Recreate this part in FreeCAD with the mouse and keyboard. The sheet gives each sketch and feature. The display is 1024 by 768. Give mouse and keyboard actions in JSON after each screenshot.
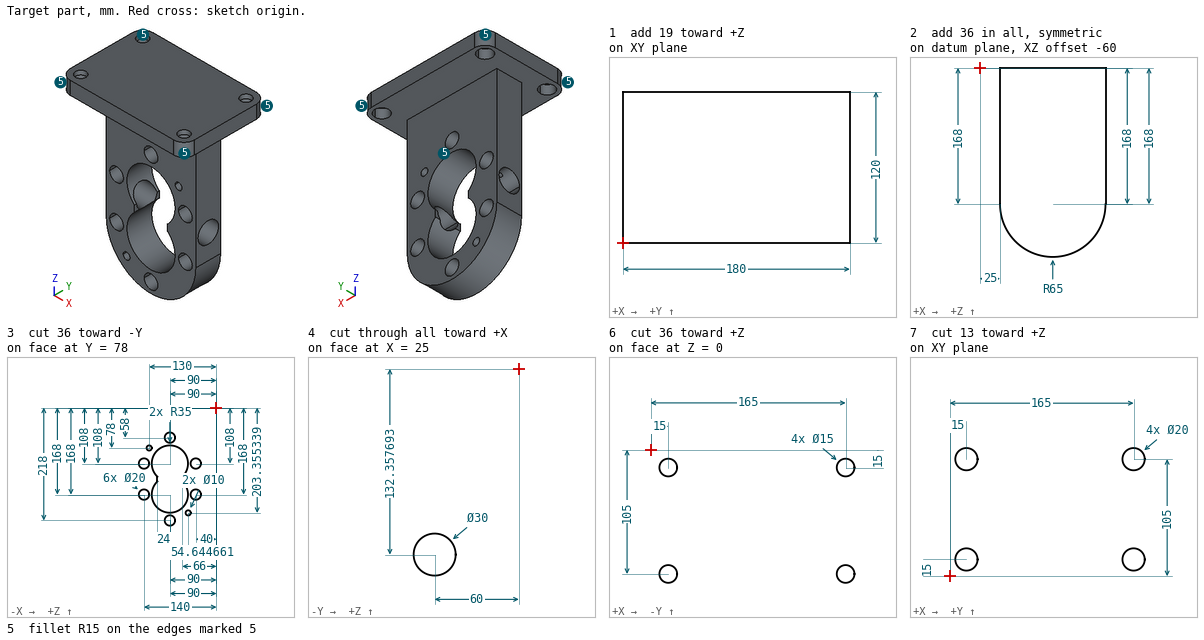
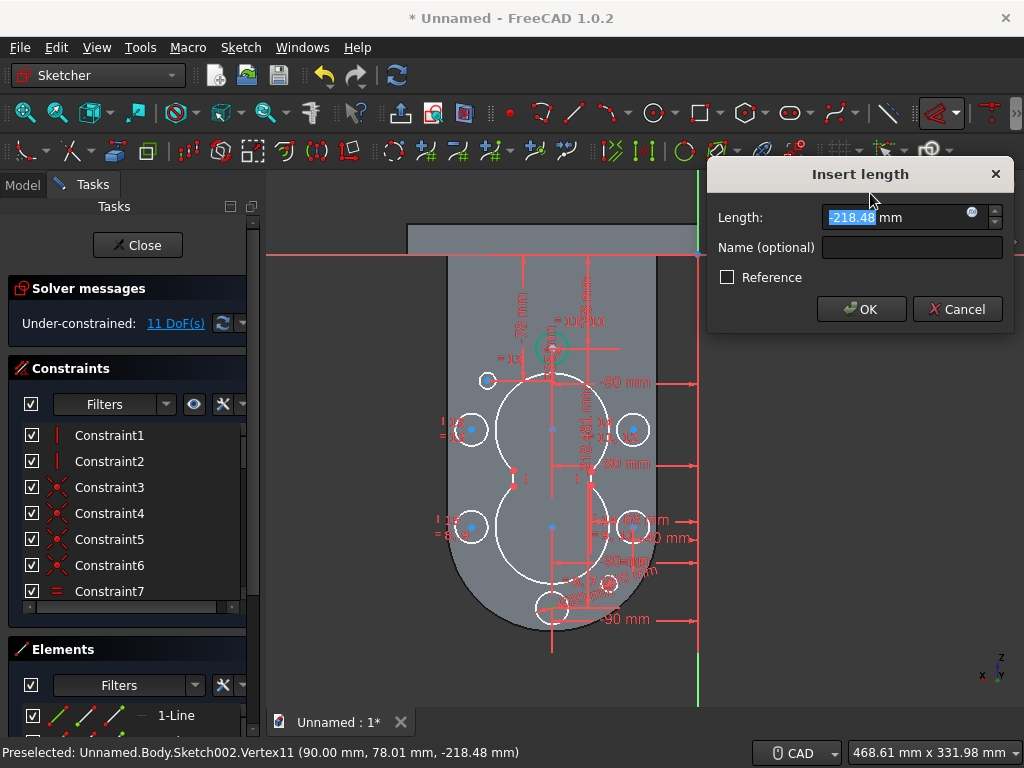
{"action": "type", "text": "-218"}
{"action": "key", "text": "Return"}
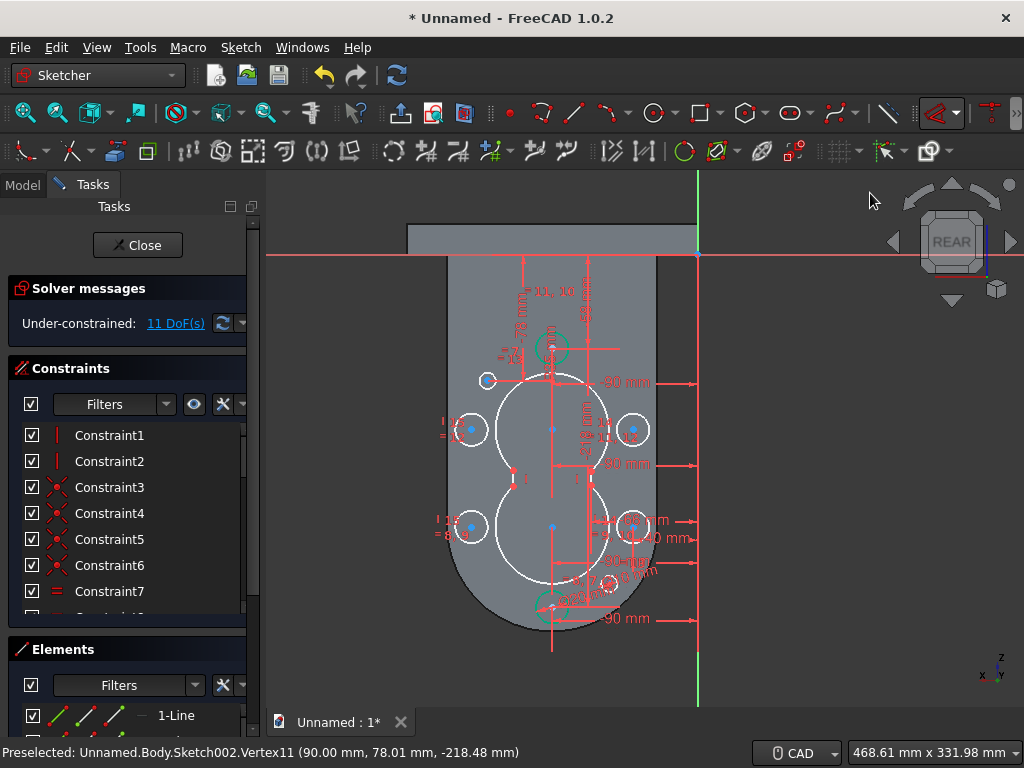
{"action": "left_click", "coordinate": [472, 527]}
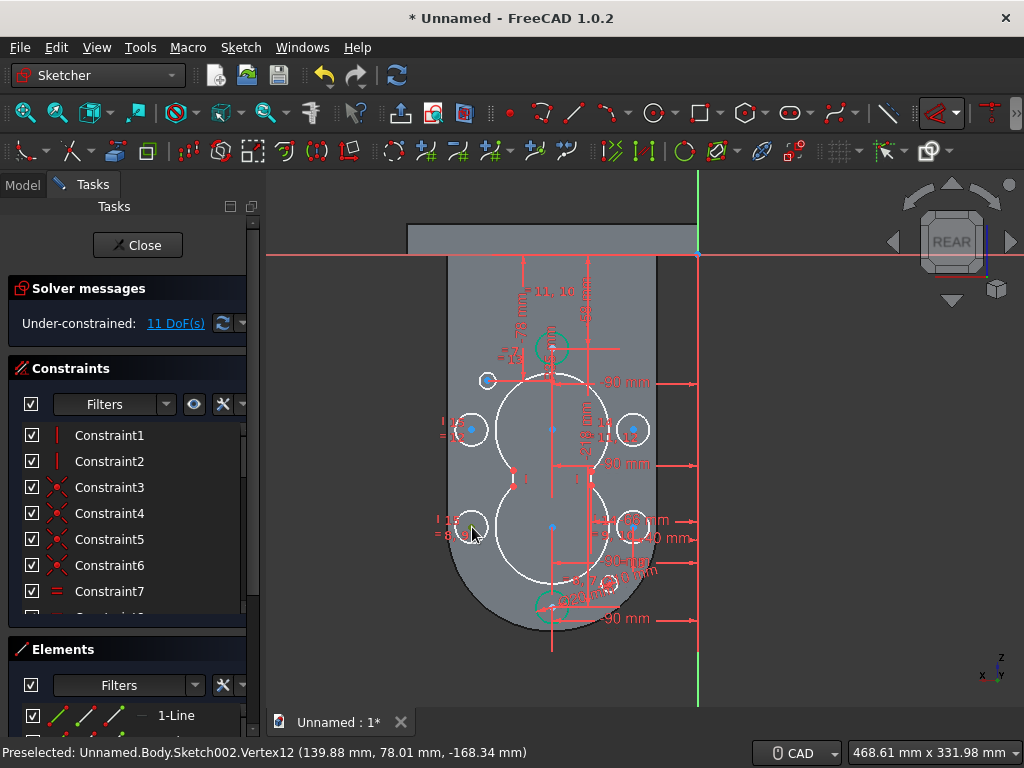
{"action": "left_click", "coordinate": [958, 114]}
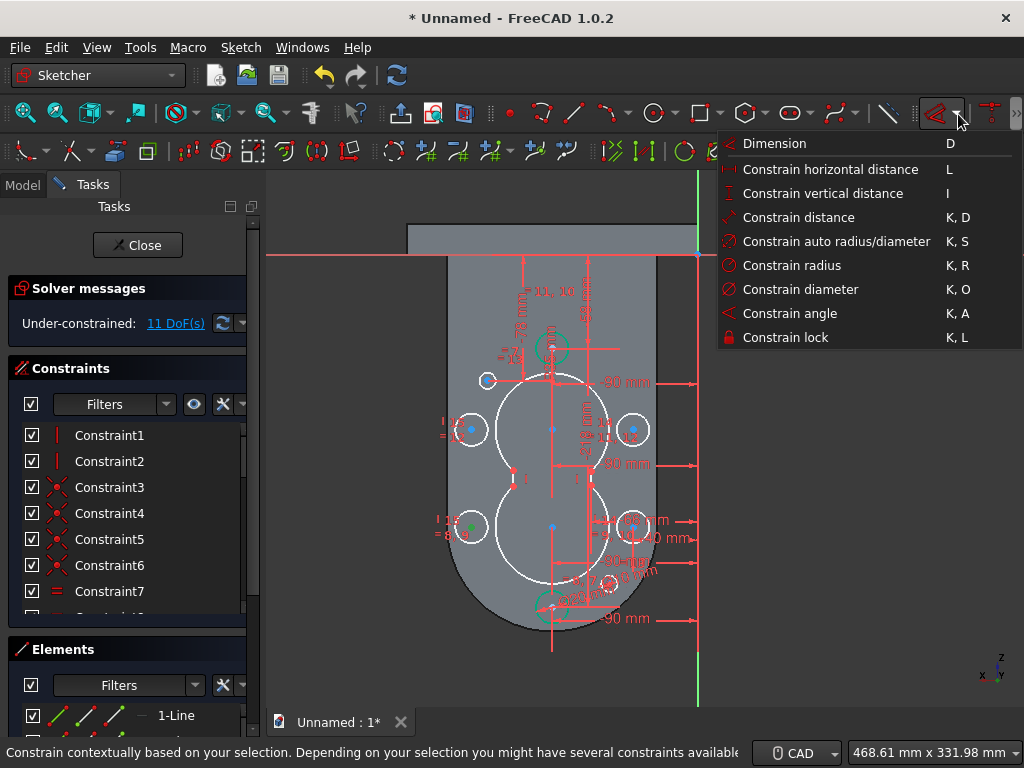
{"action": "left_click", "coordinate": [870, 169]}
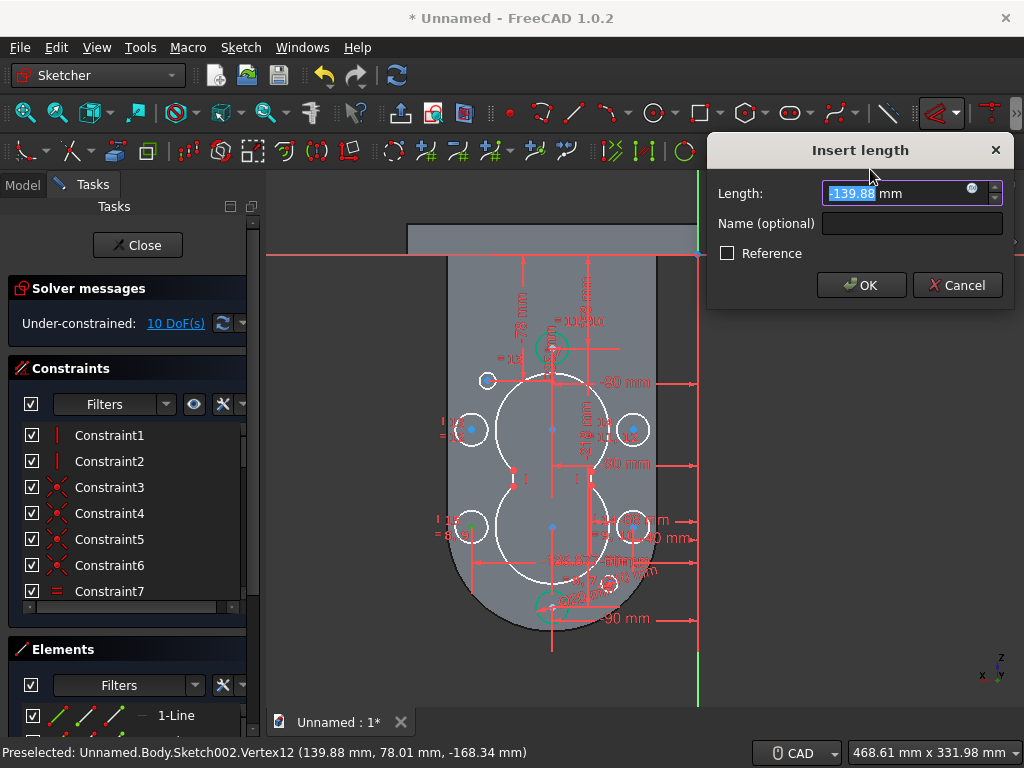
{"action": "type", "text": "-140"}
{"action": "key", "text": "Return"}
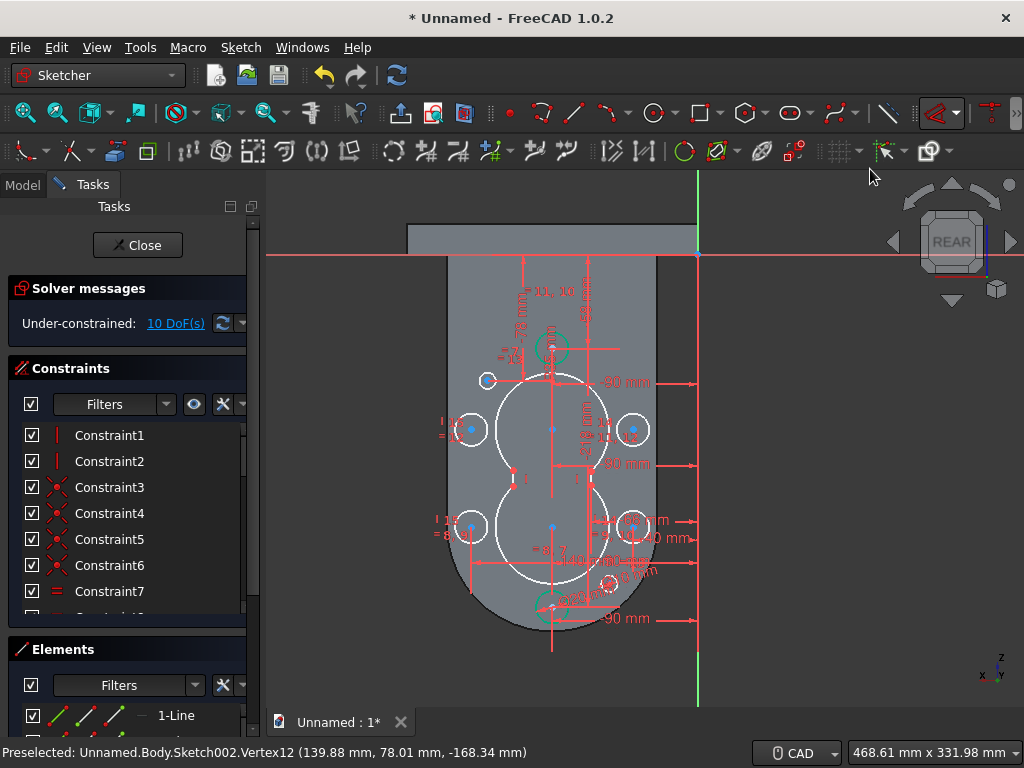
{"action": "left_click", "coordinate": [471, 527]}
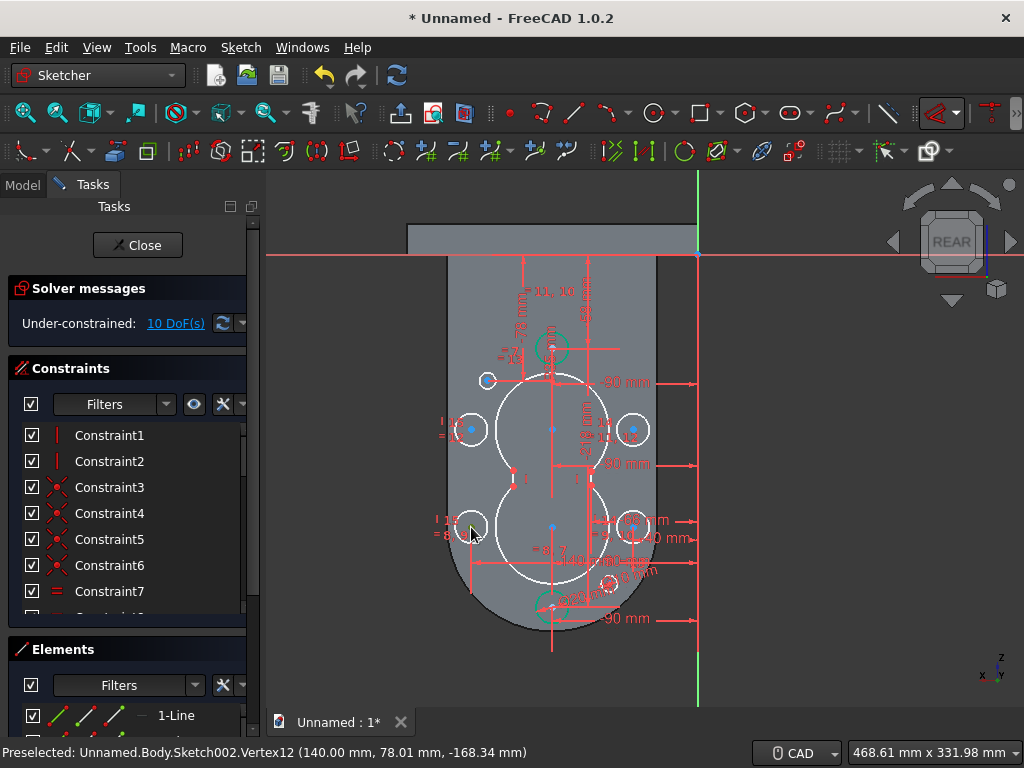
{"action": "key", "text": "i"}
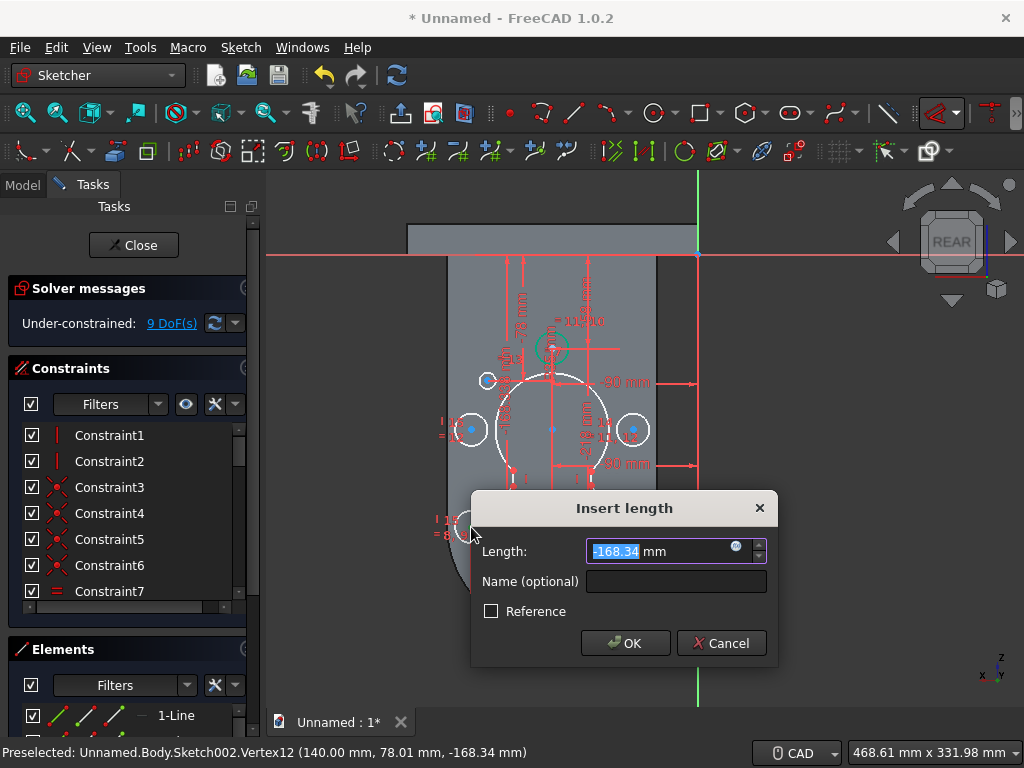
{"action": "type", "text": "-168"}
{"action": "key", "text": "Return"}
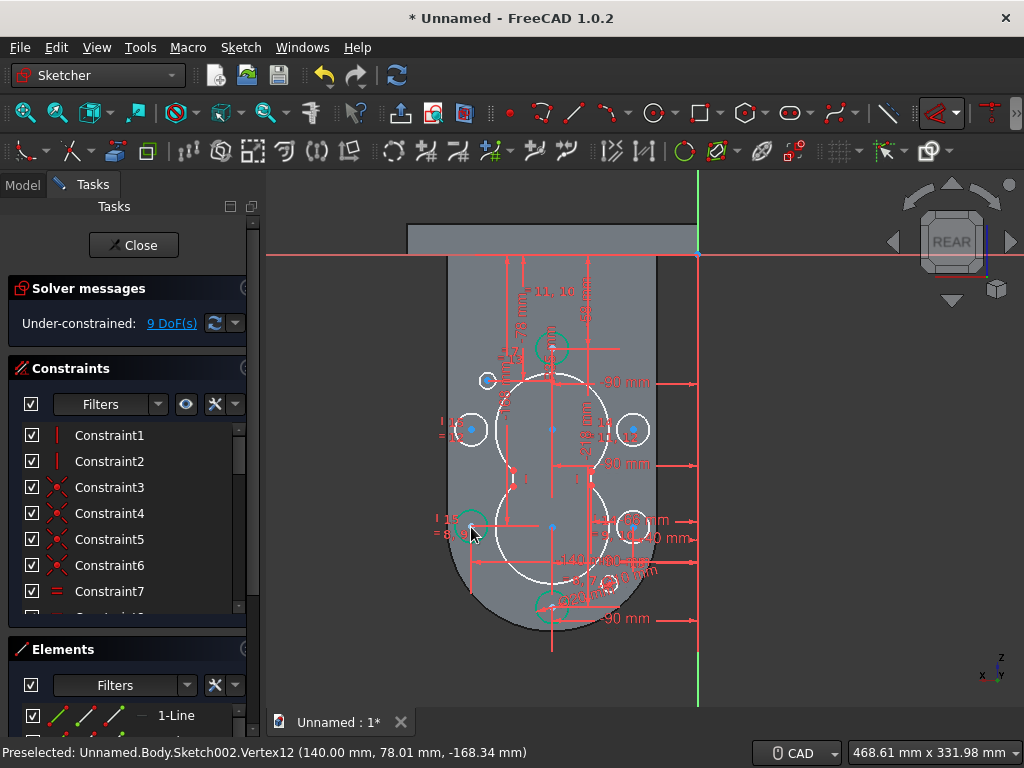
{"action": "left_click", "coordinate": [633, 527]}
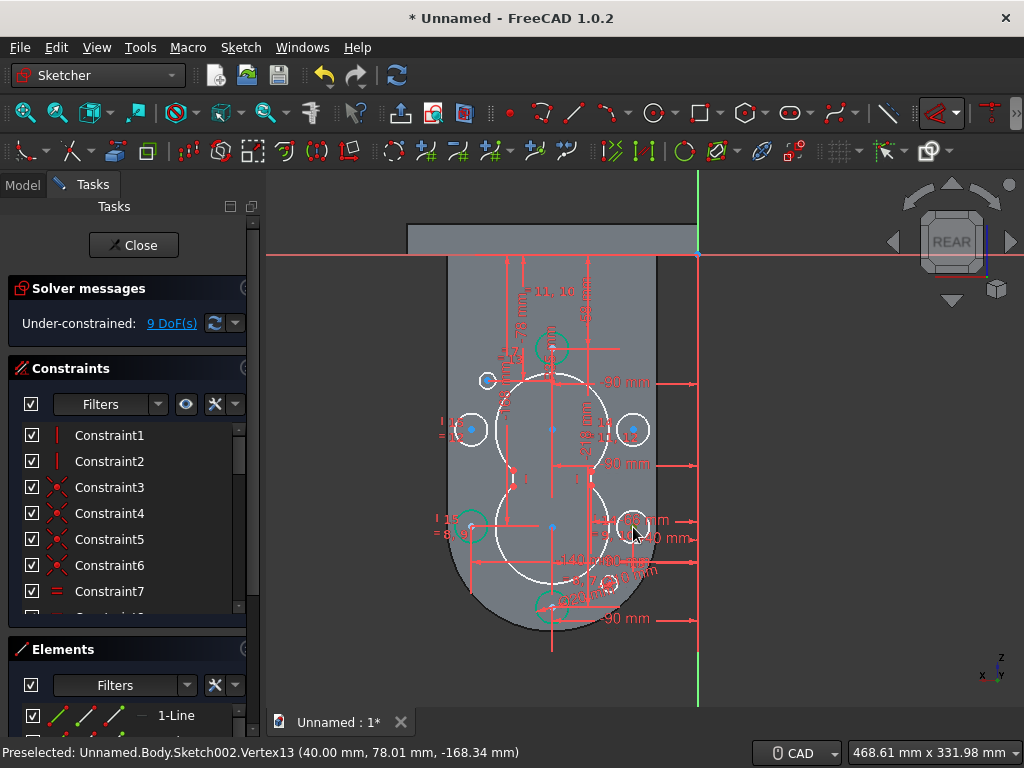
{"action": "key", "text": "i"}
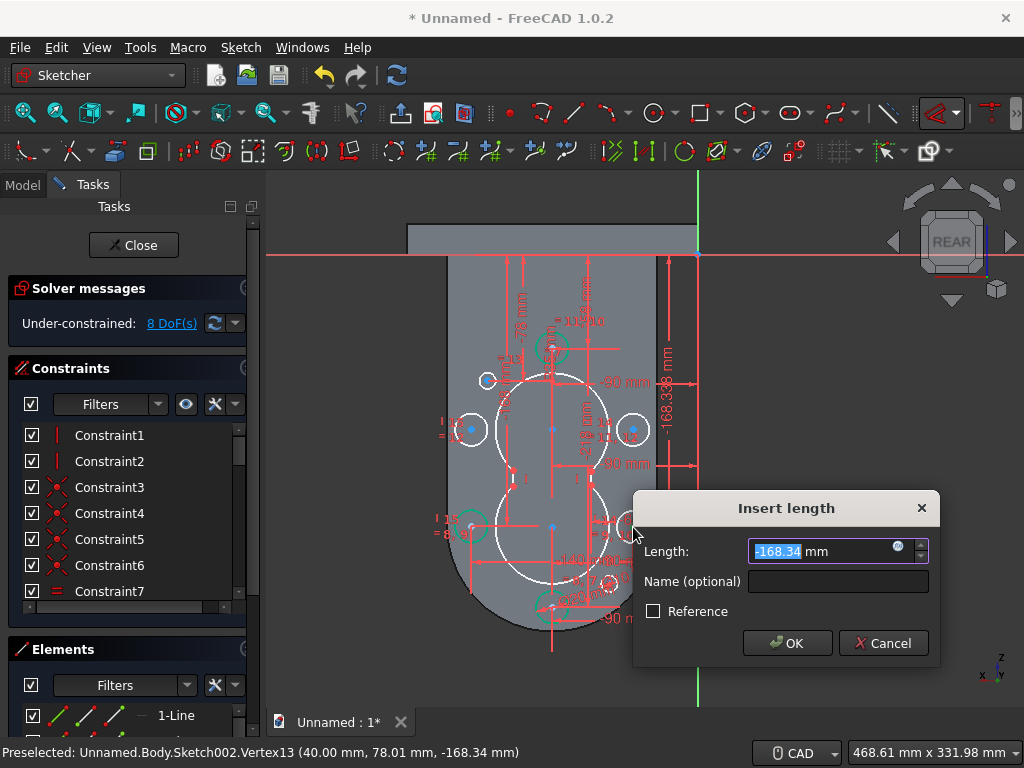
{"action": "type", "text": "-168"}
{"action": "key", "text": "Return"}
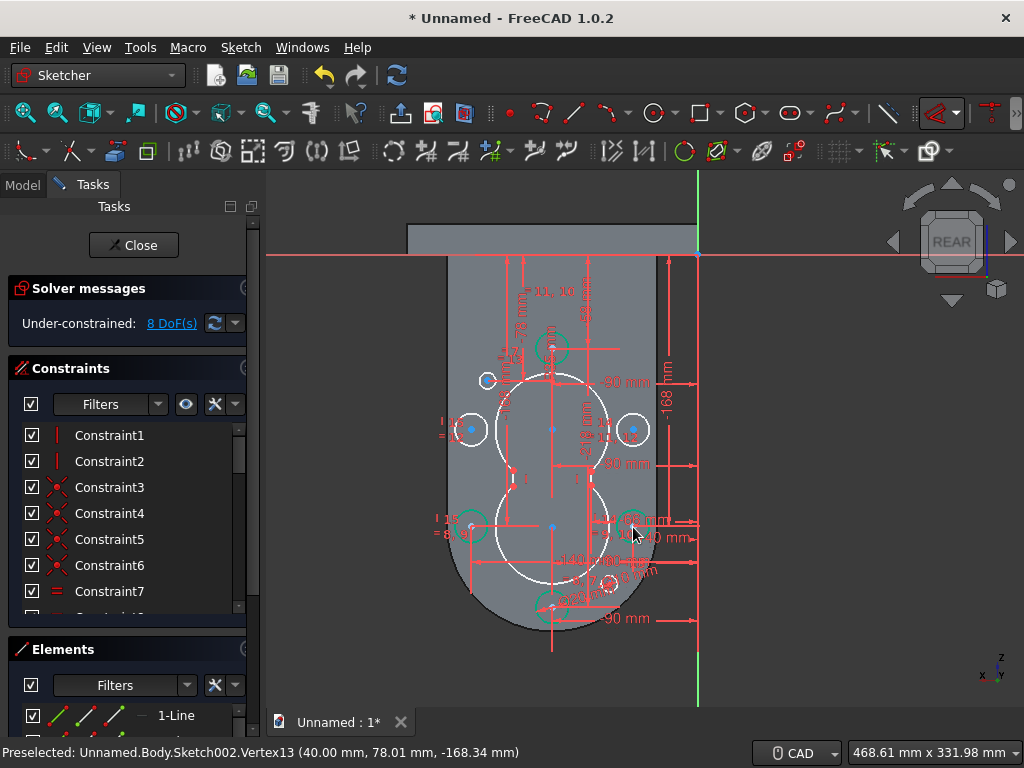
{"action": "scroll", "coordinate": [633, 430], "scroll_direction": "up", "scroll_amount": 4}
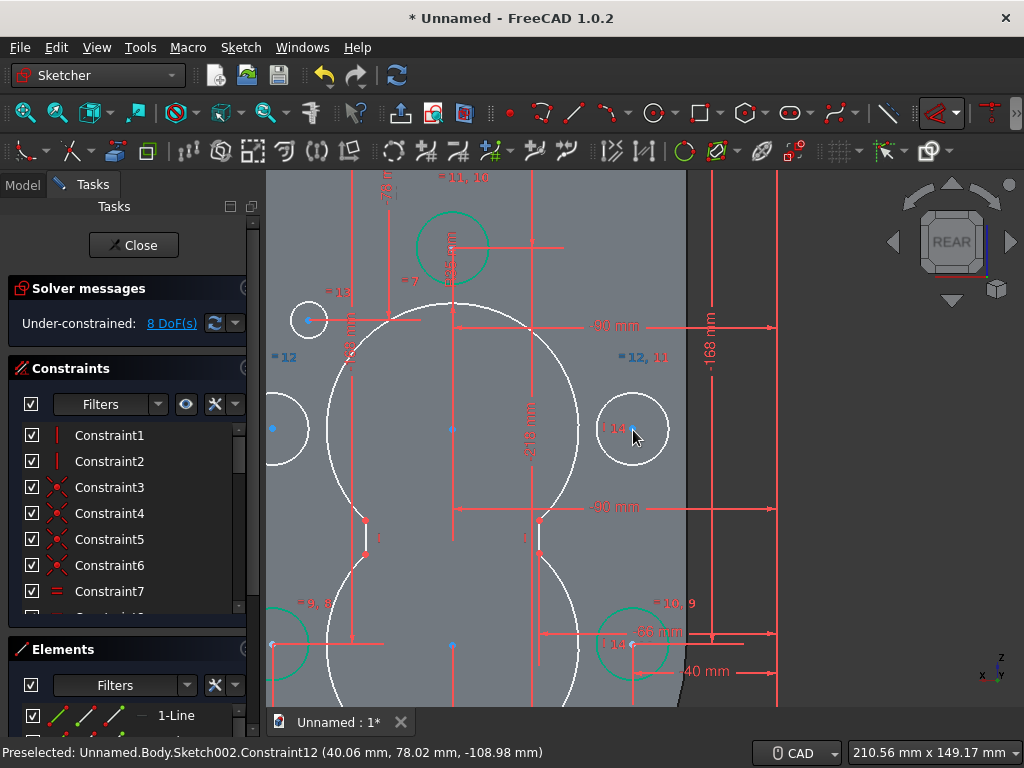
{"action": "left_click", "coordinate": [633, 429]}